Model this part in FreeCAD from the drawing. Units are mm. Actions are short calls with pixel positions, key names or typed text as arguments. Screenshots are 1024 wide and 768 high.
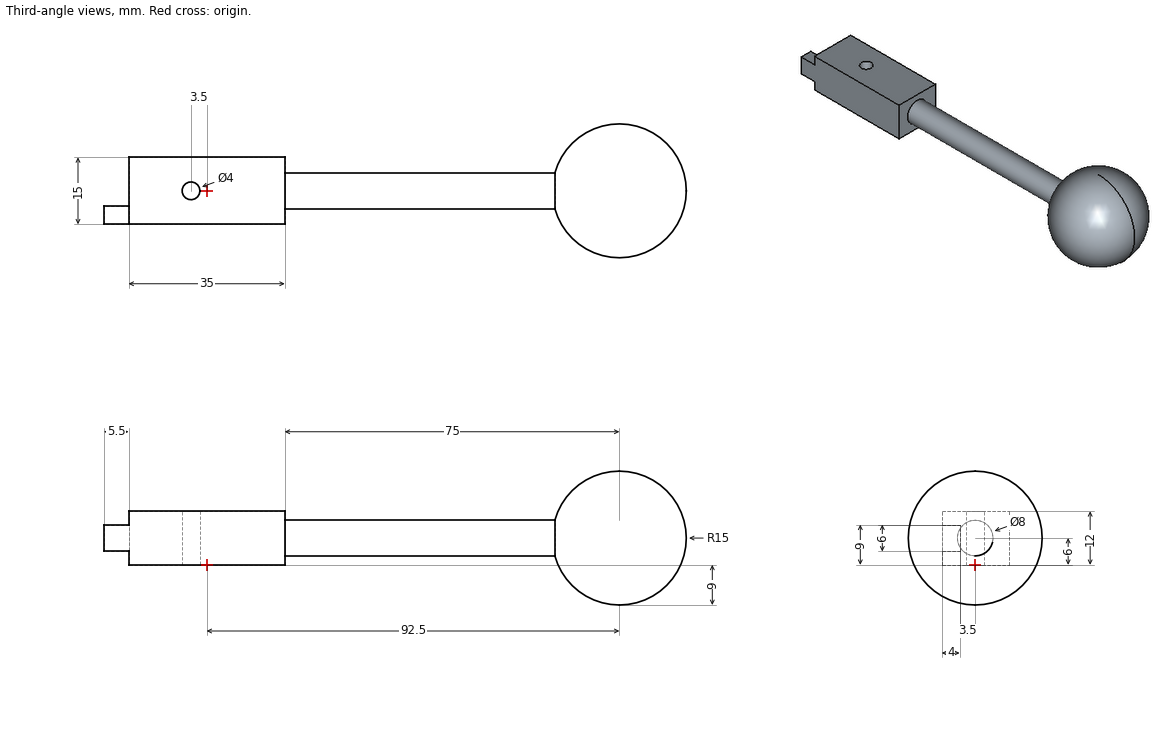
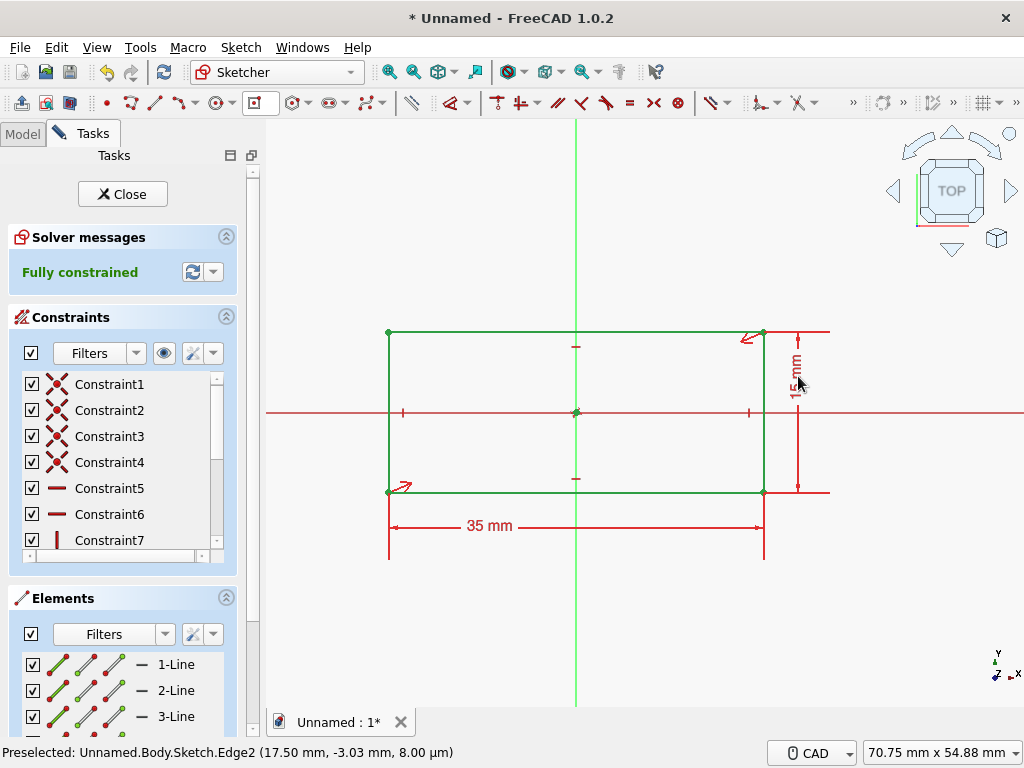
click(123, 194)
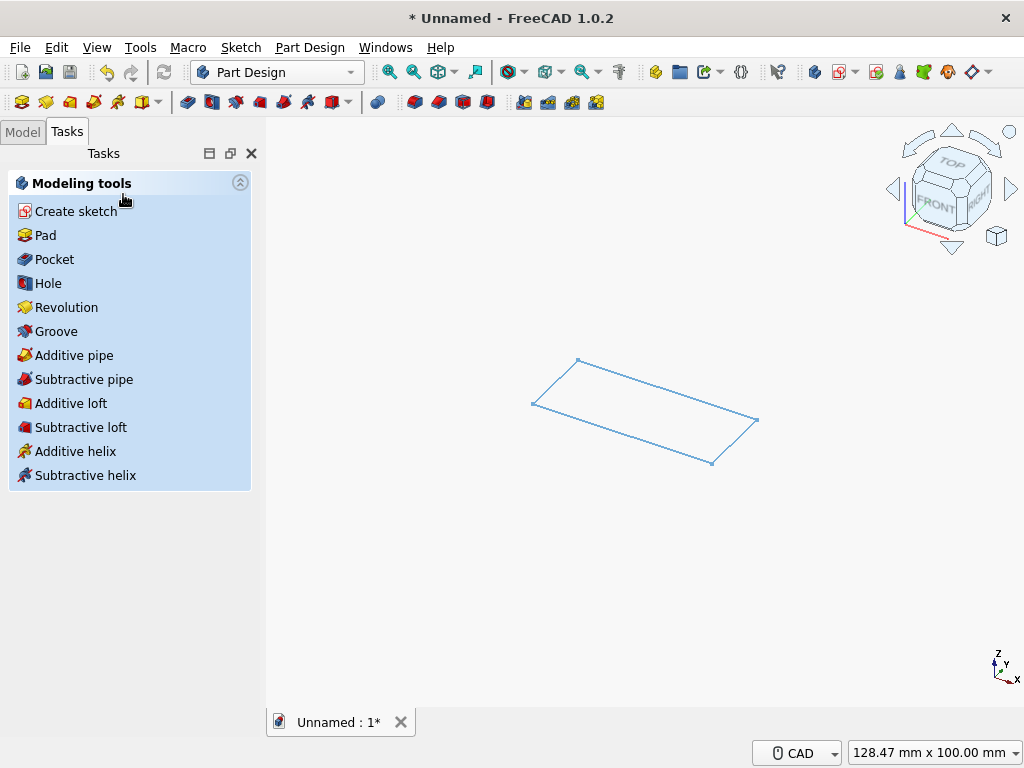
click(22, 102)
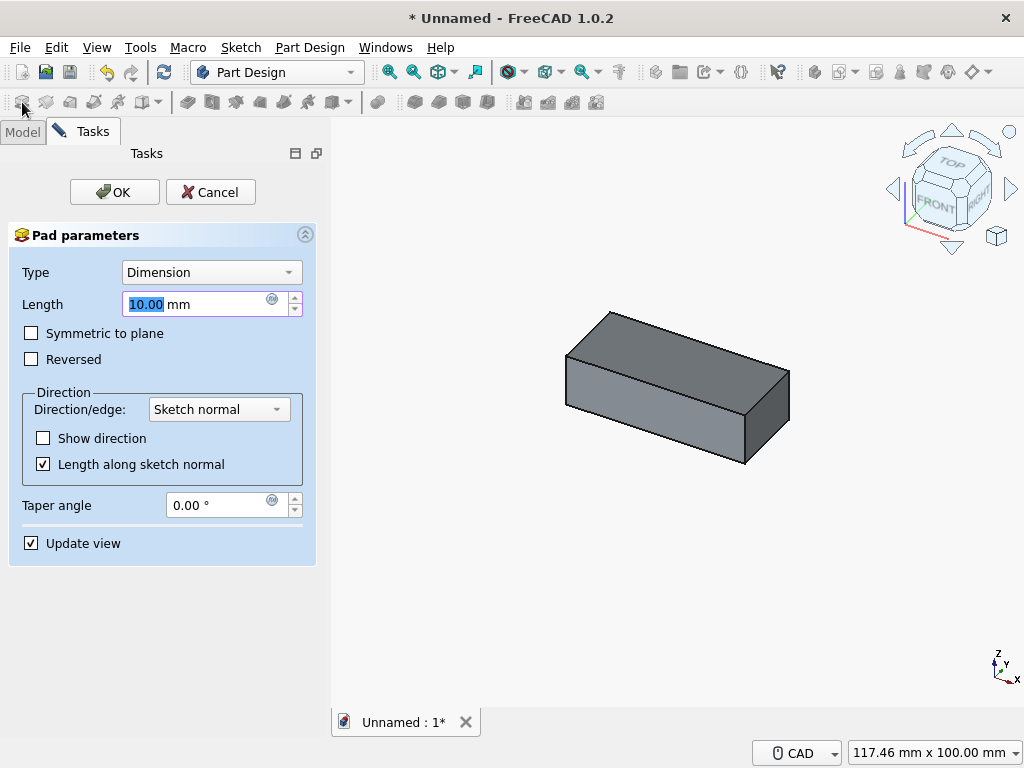
text(12)
key(Tab)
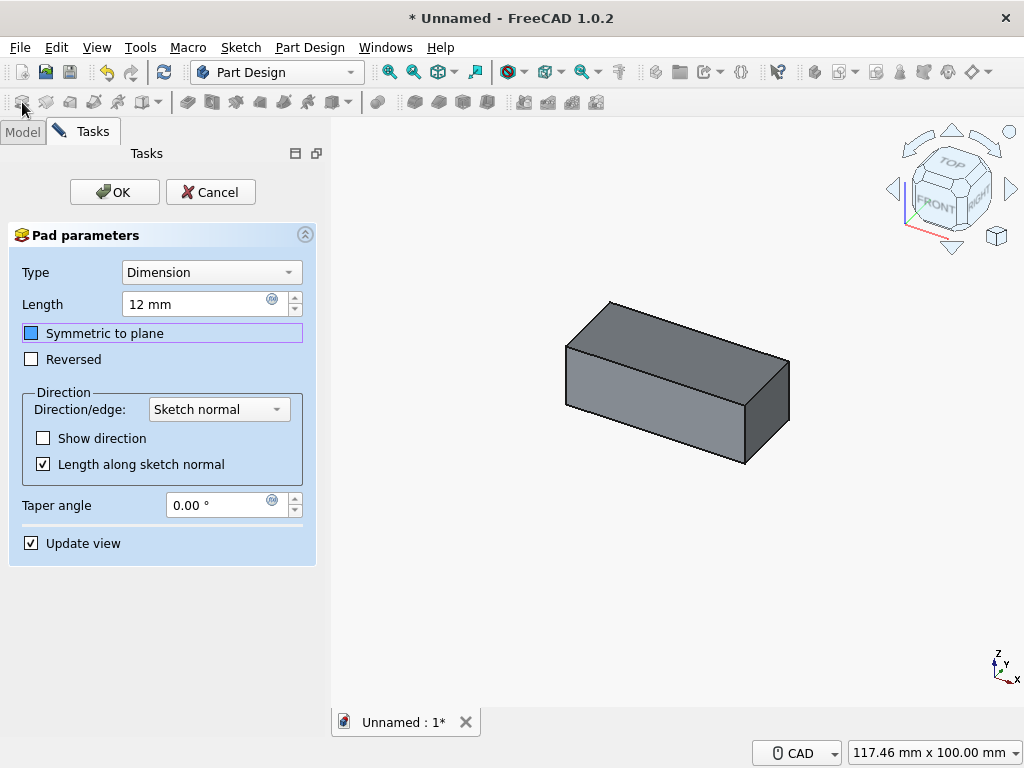
click(115, 192)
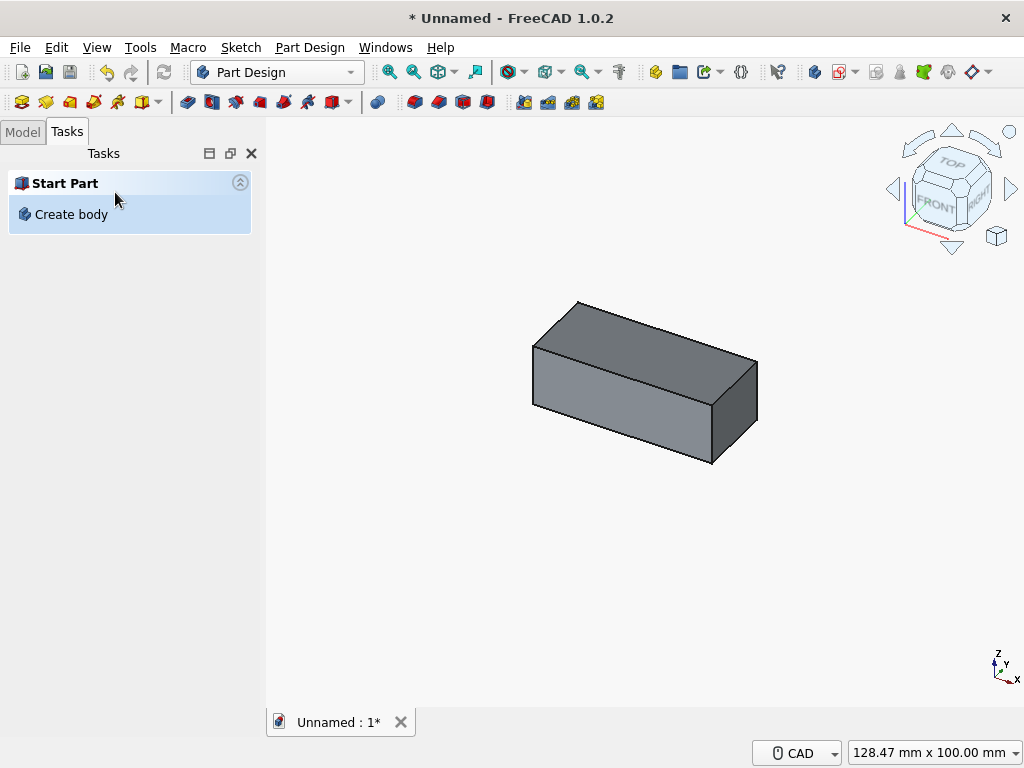
click(390, 72)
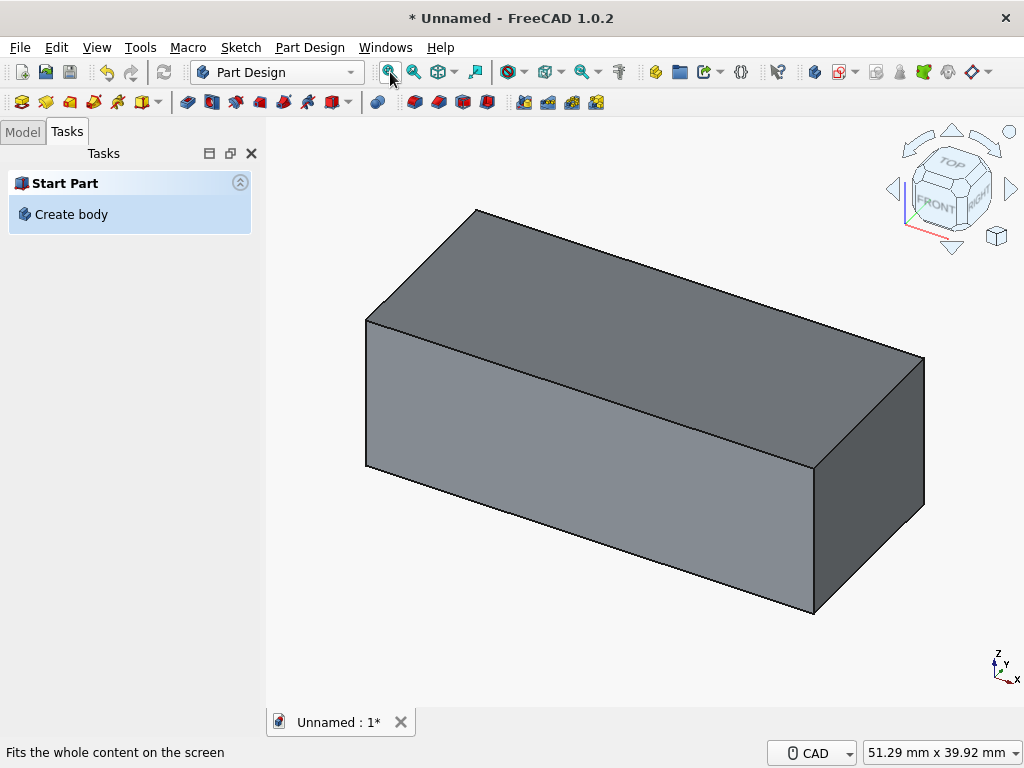
key(6)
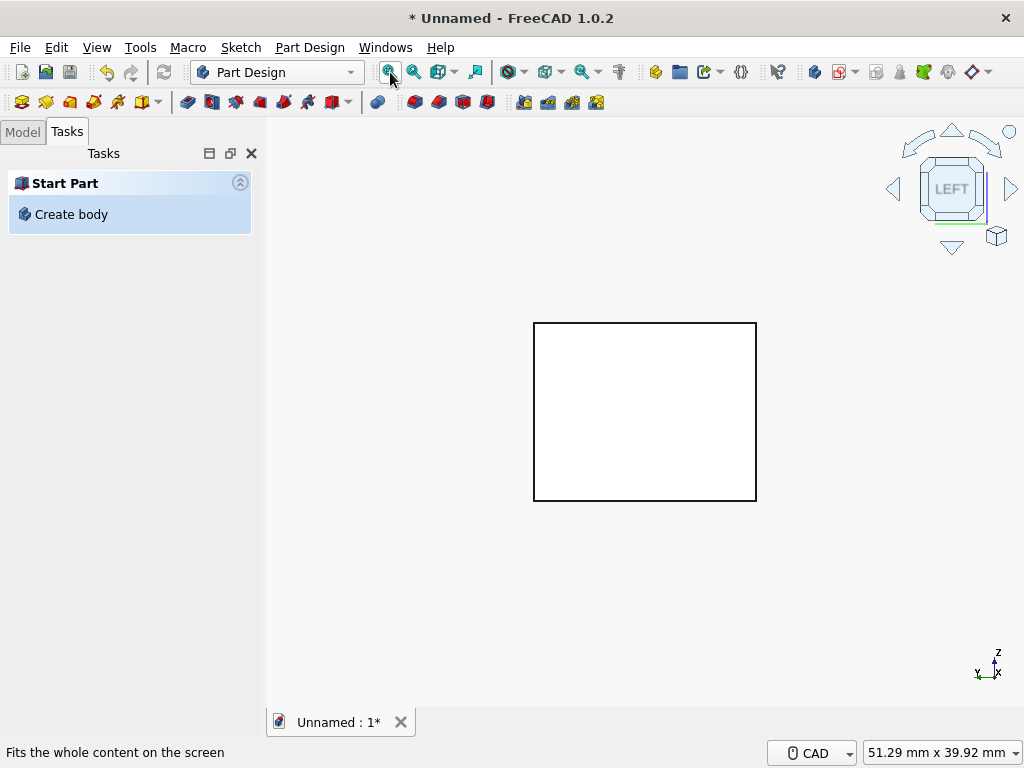
click(390, 72)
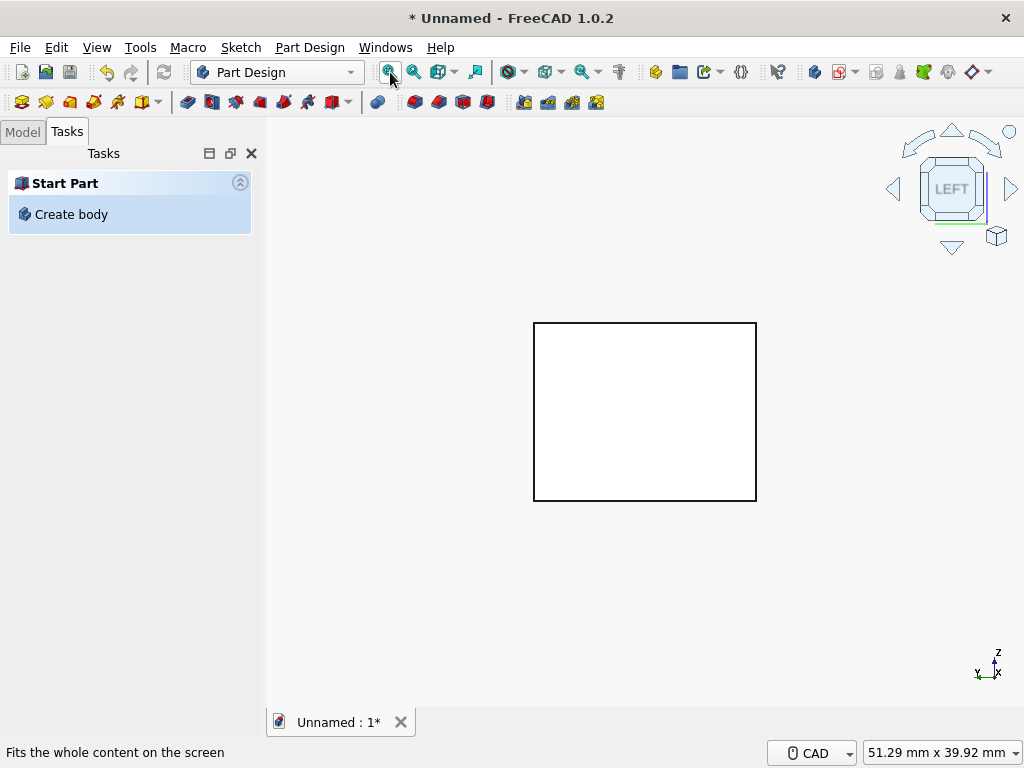
click(645, 411)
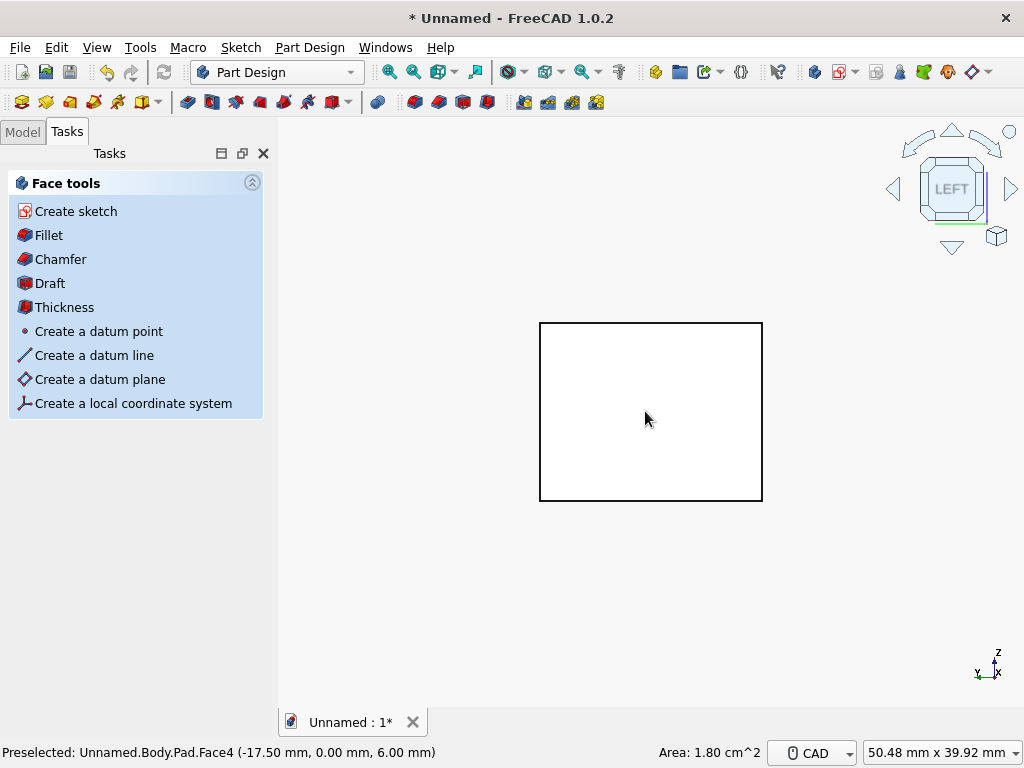
click(840, 72)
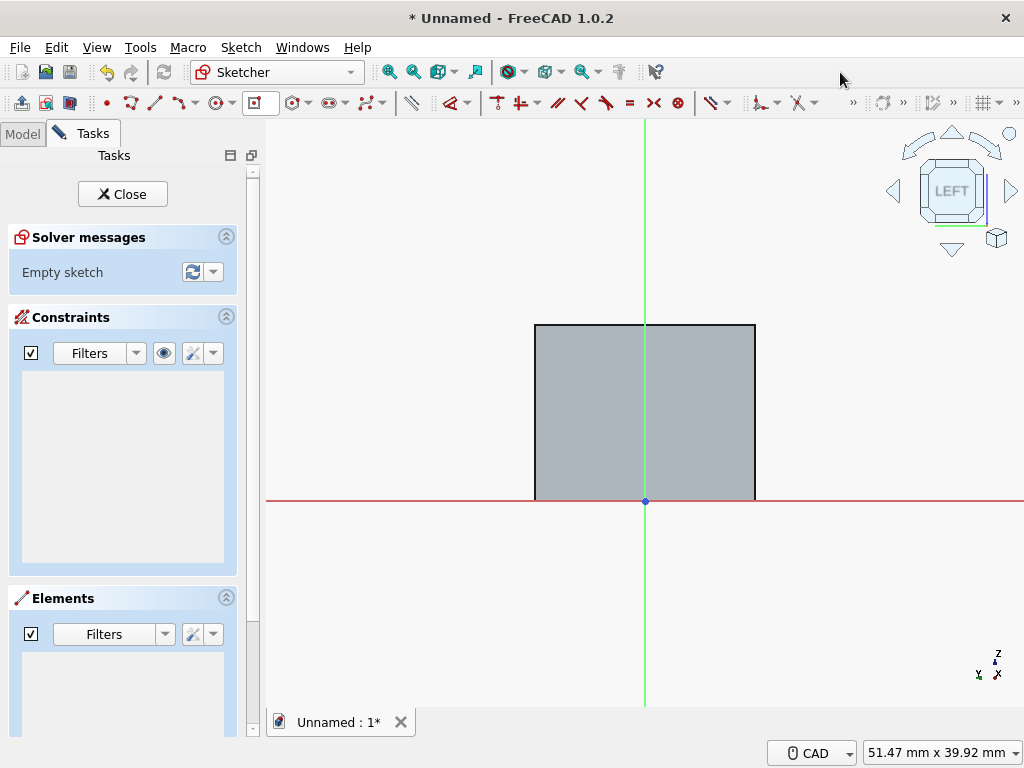
scroll(772, 448, up, 5)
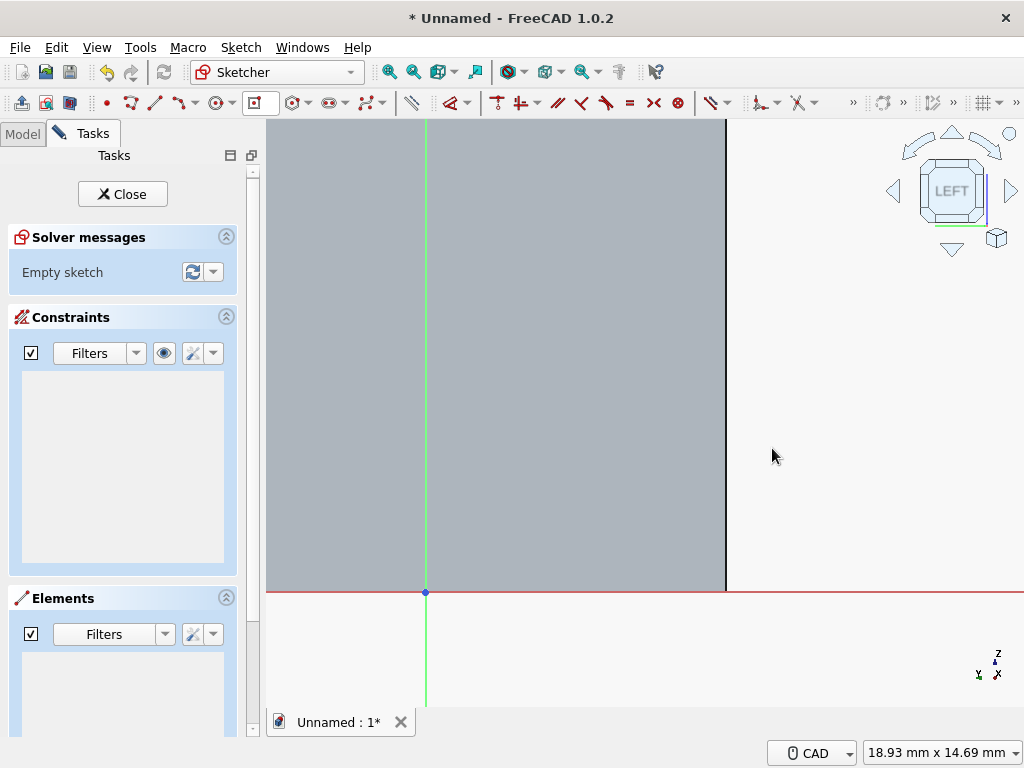
key(g)
key(r)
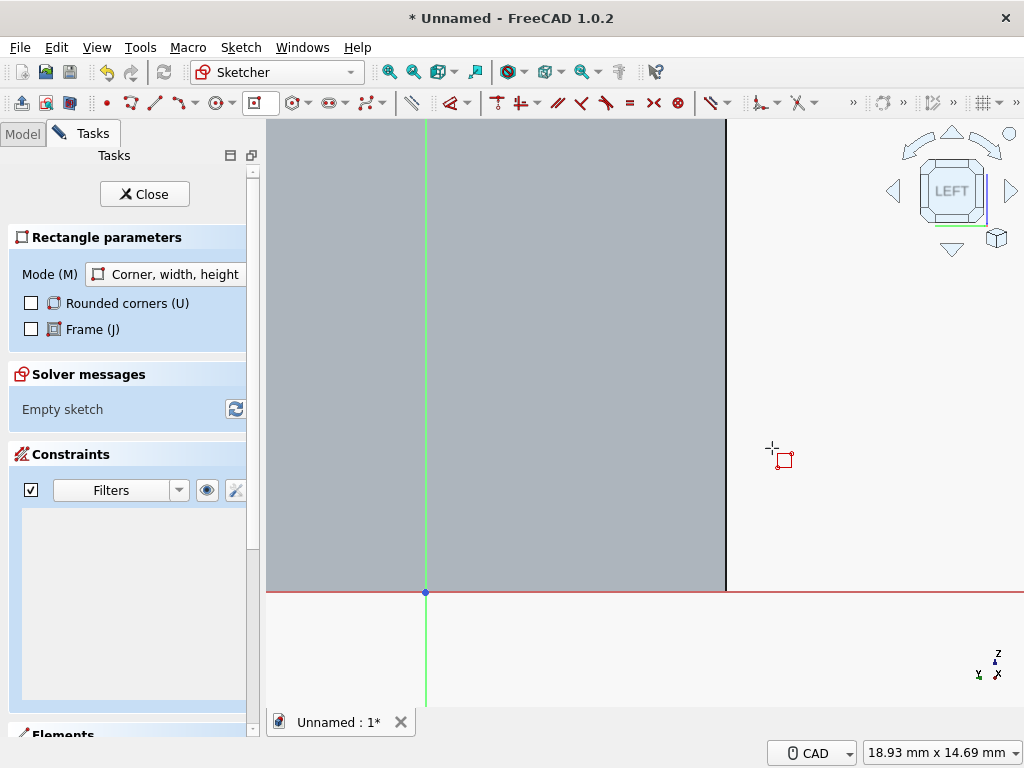
click(566, 232)
click(726, 472)
key(Escape)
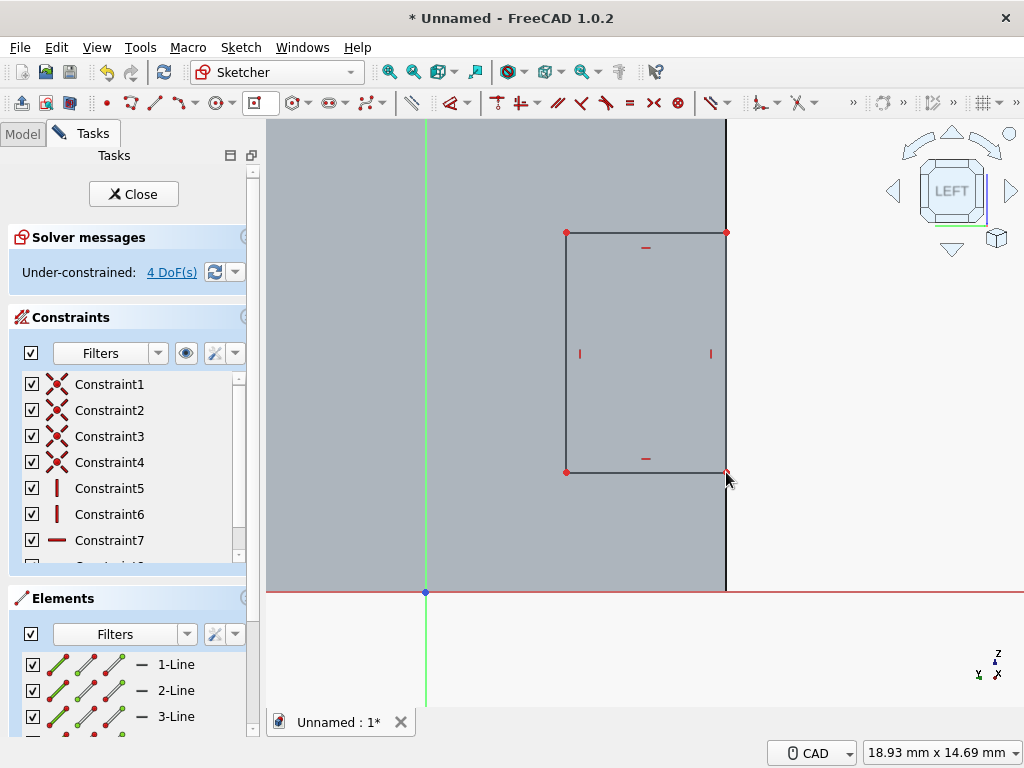
click(450, 104)